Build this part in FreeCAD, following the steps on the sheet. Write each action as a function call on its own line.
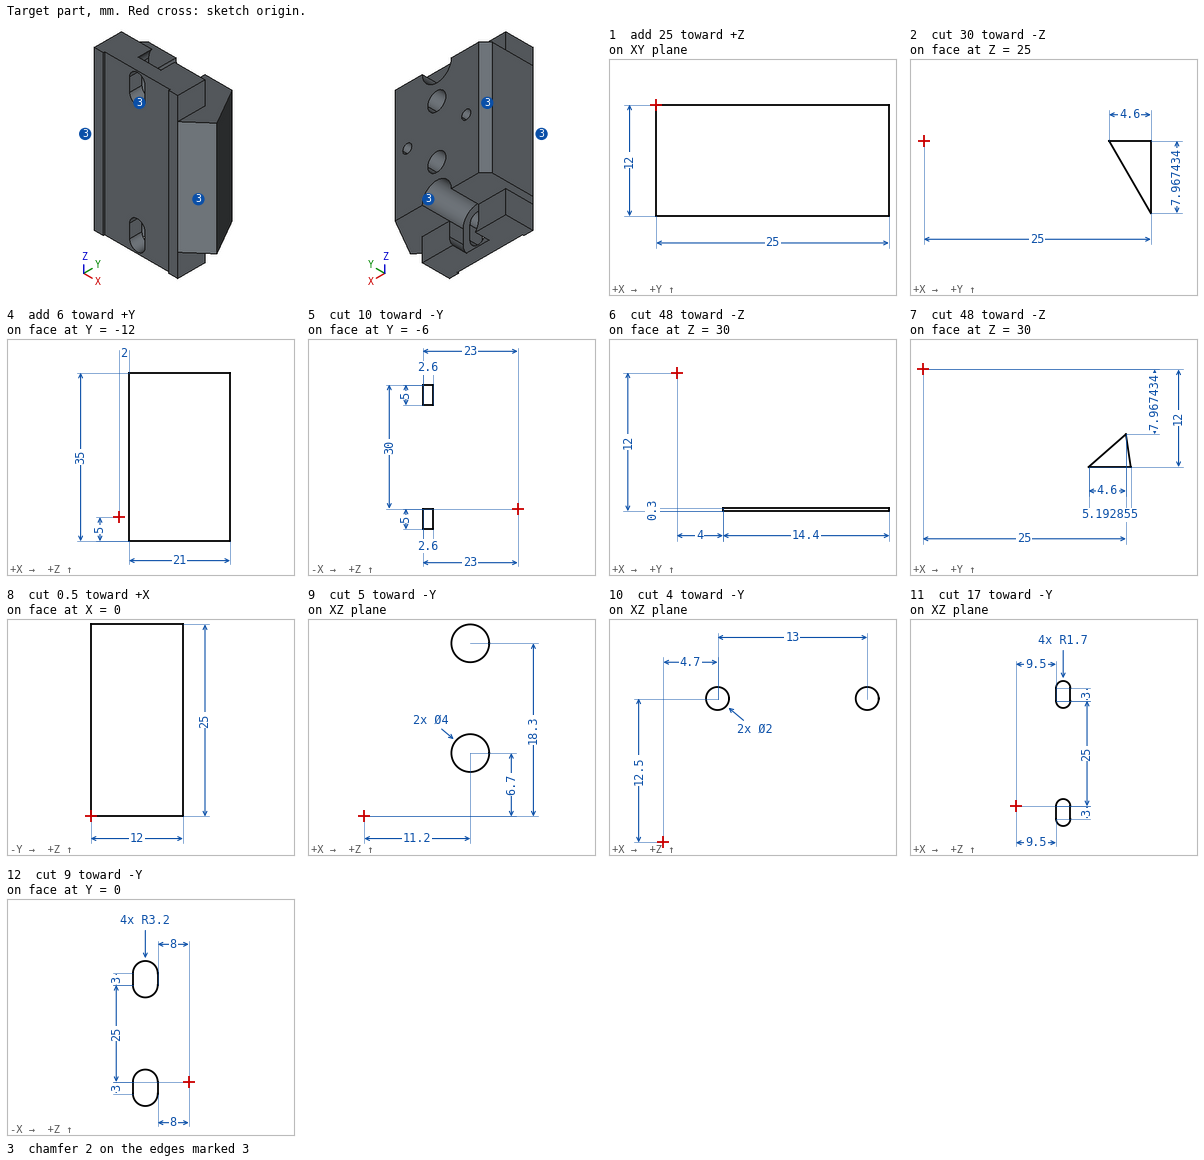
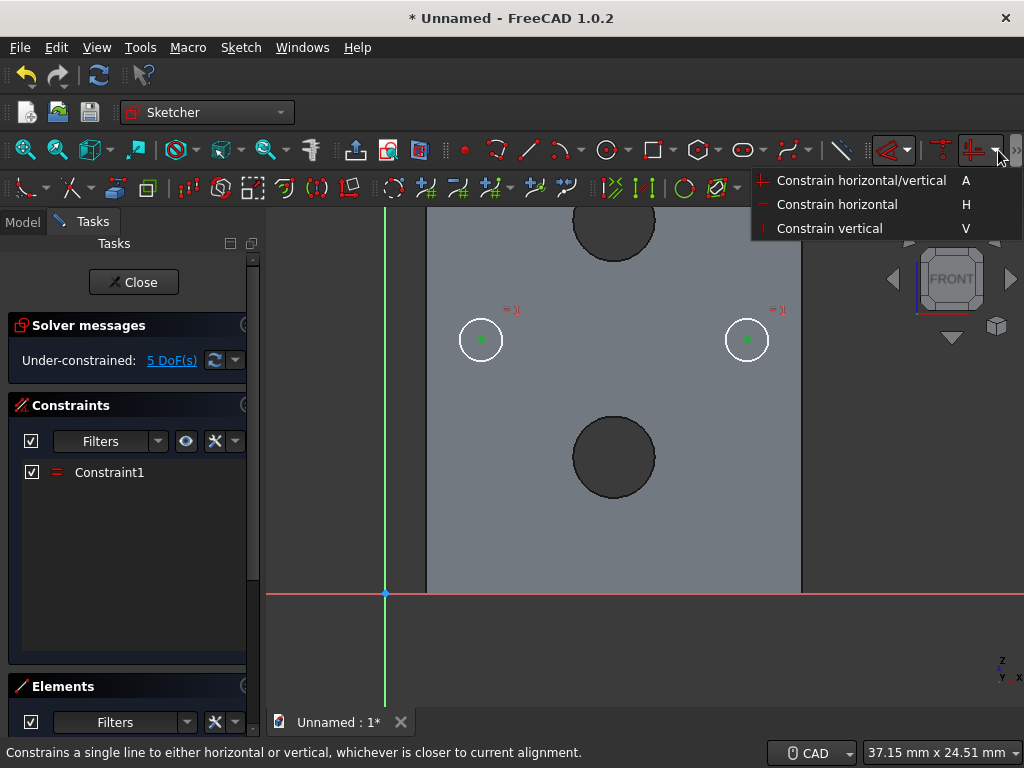
click(887, 204)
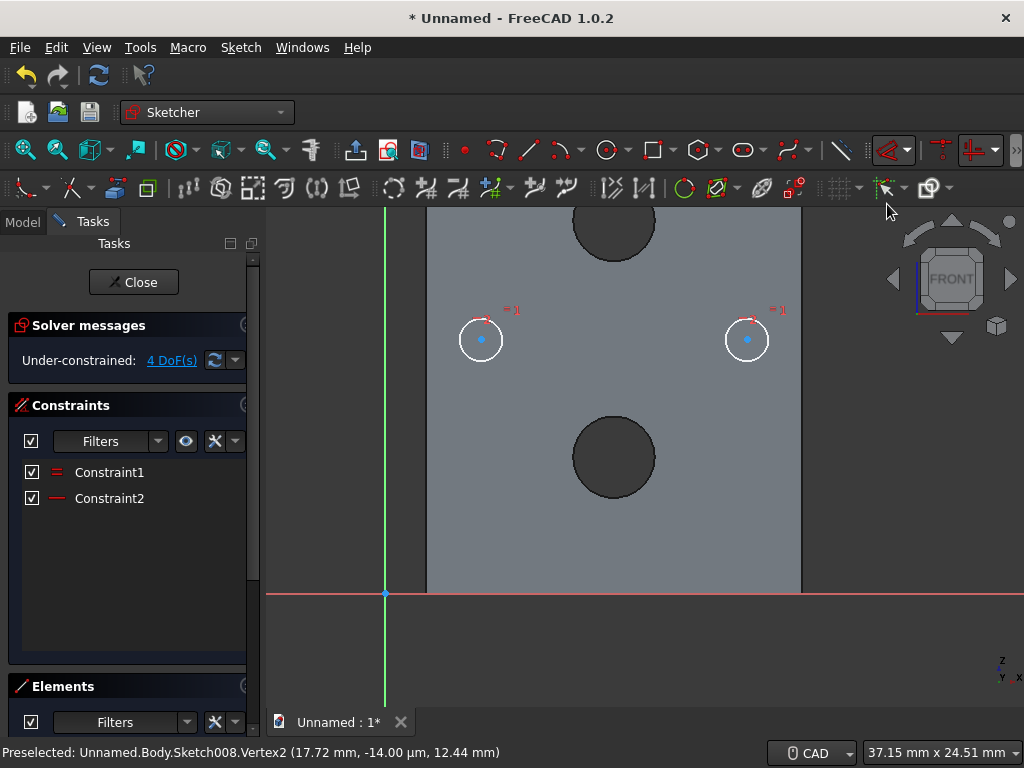
click(496, 325)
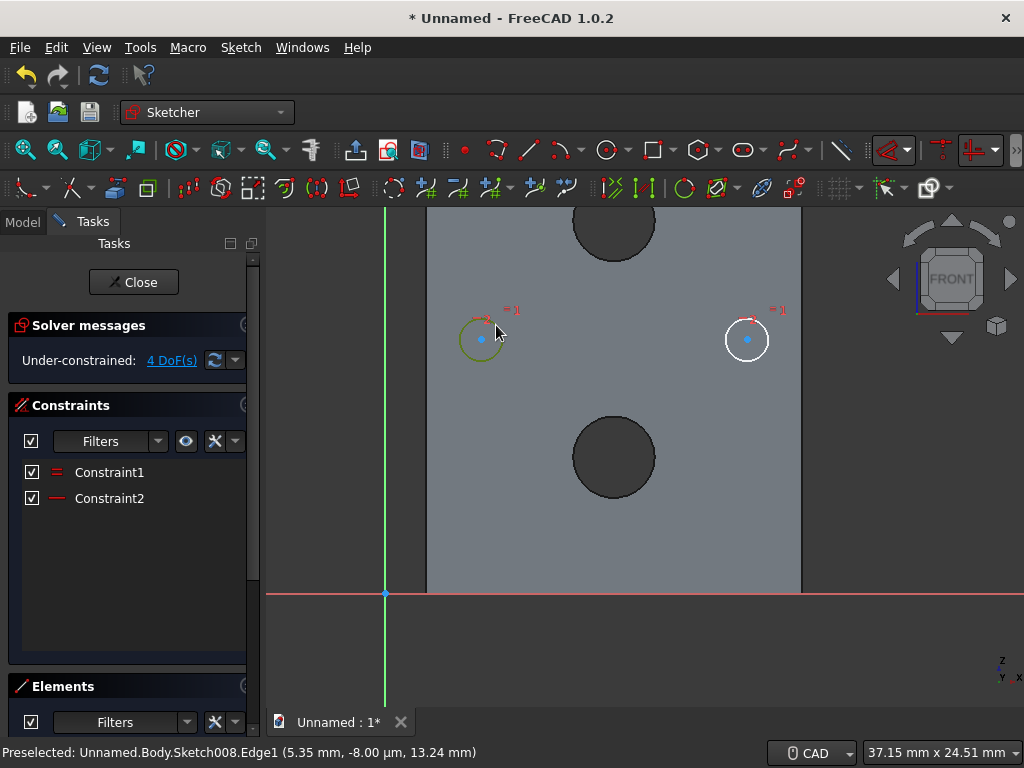
click(910, 150)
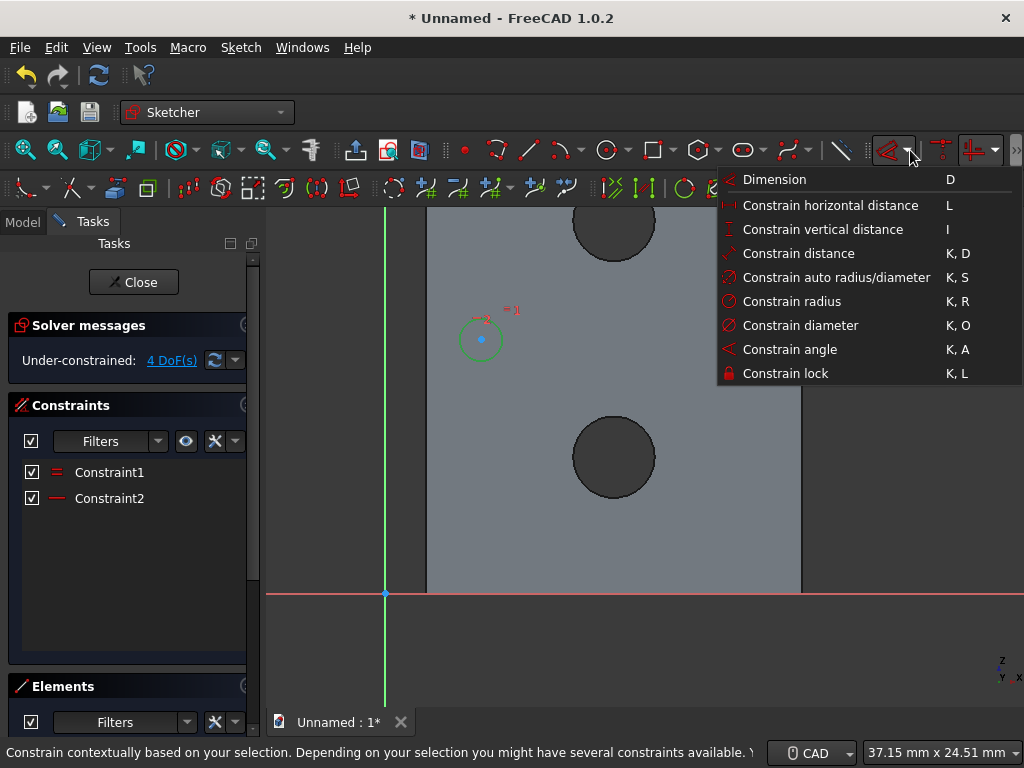
click(870, 325)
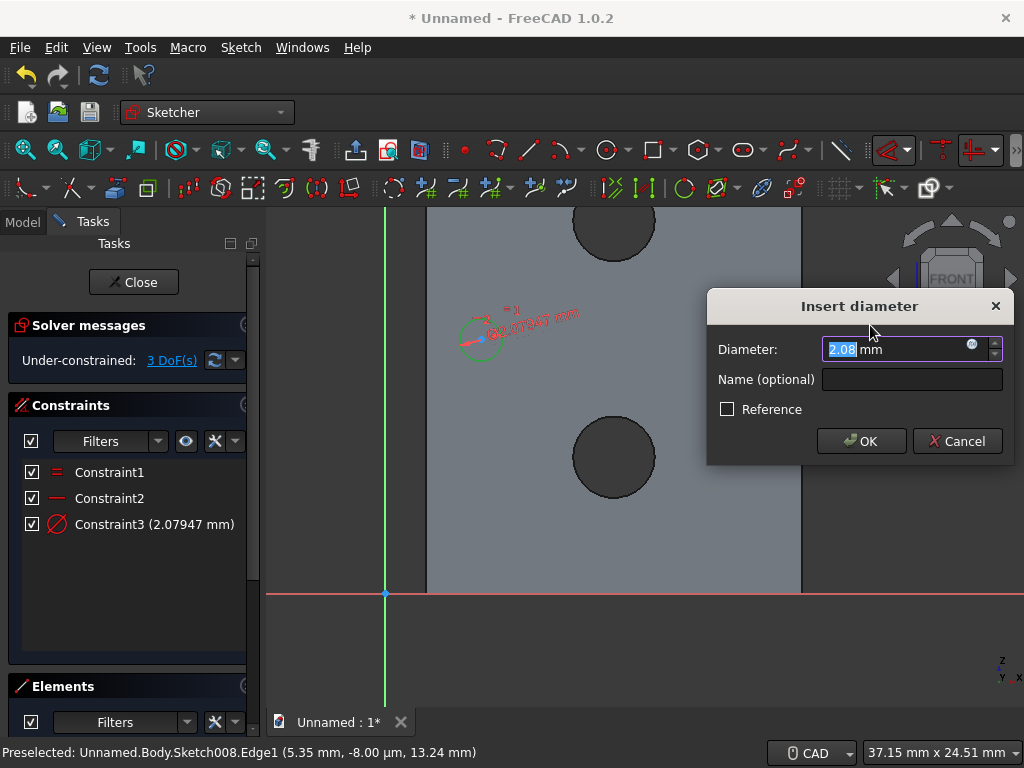
text(2)
key(Return)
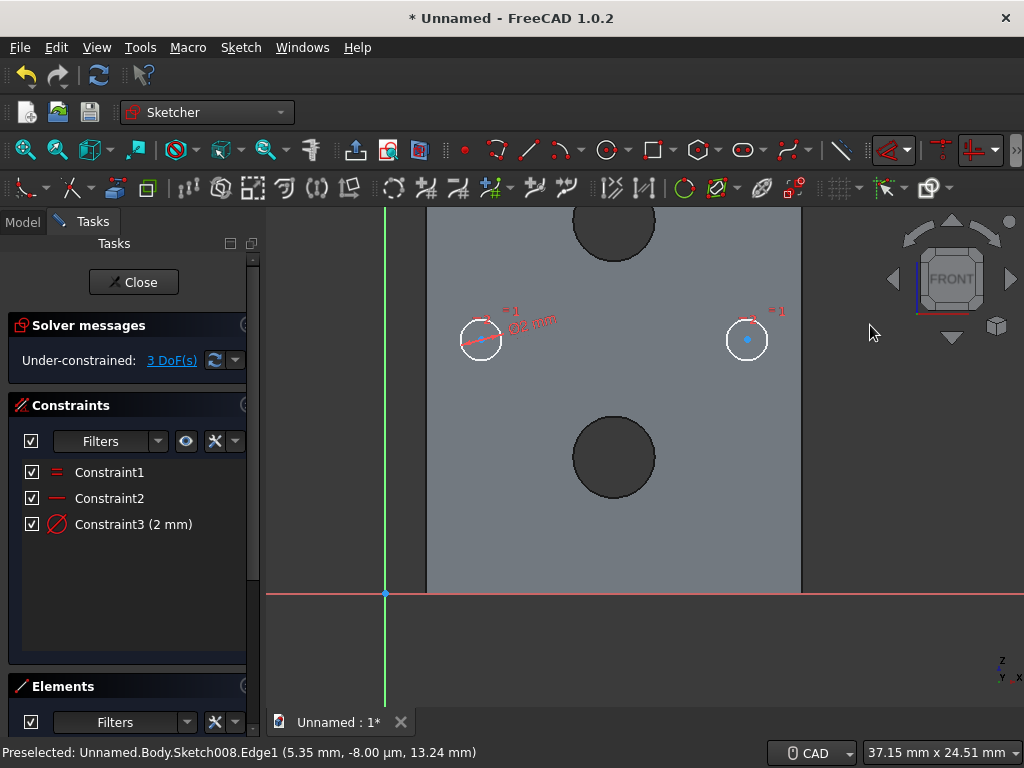
click(481, 340)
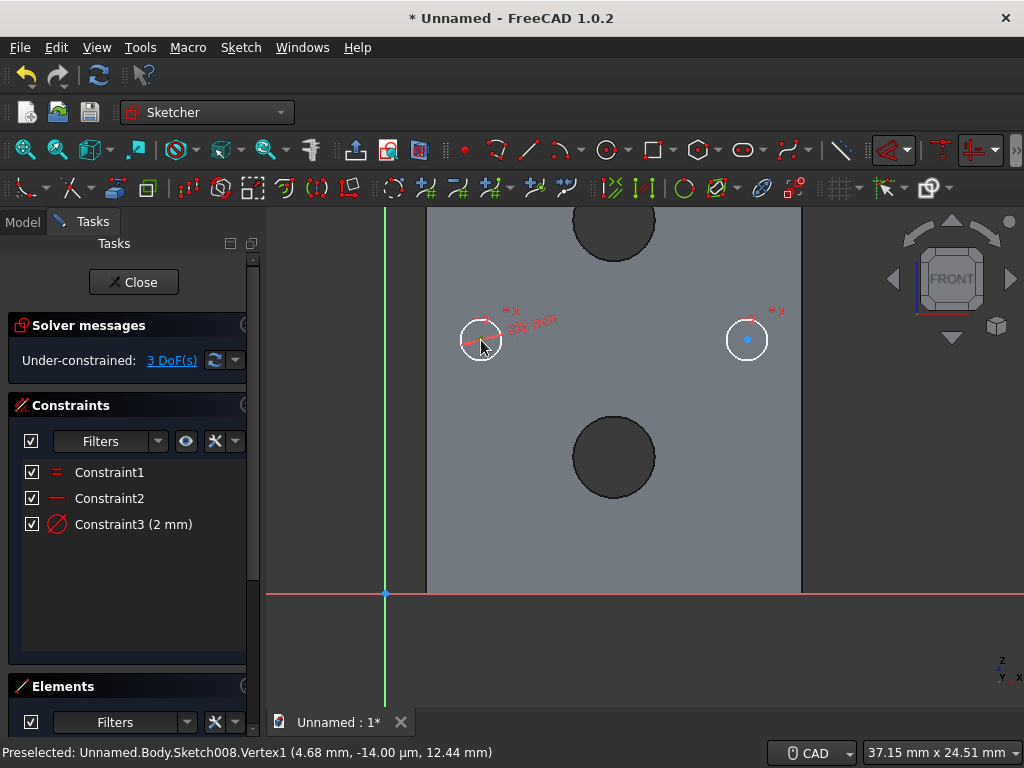
click(910, 150)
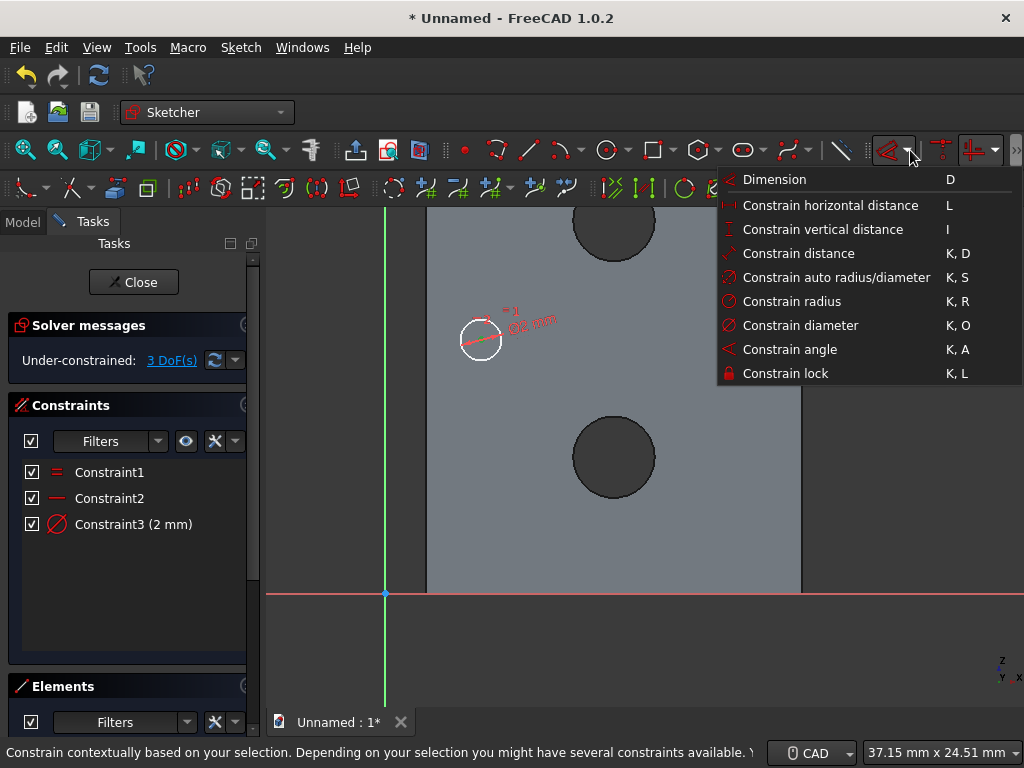
click(870, 205)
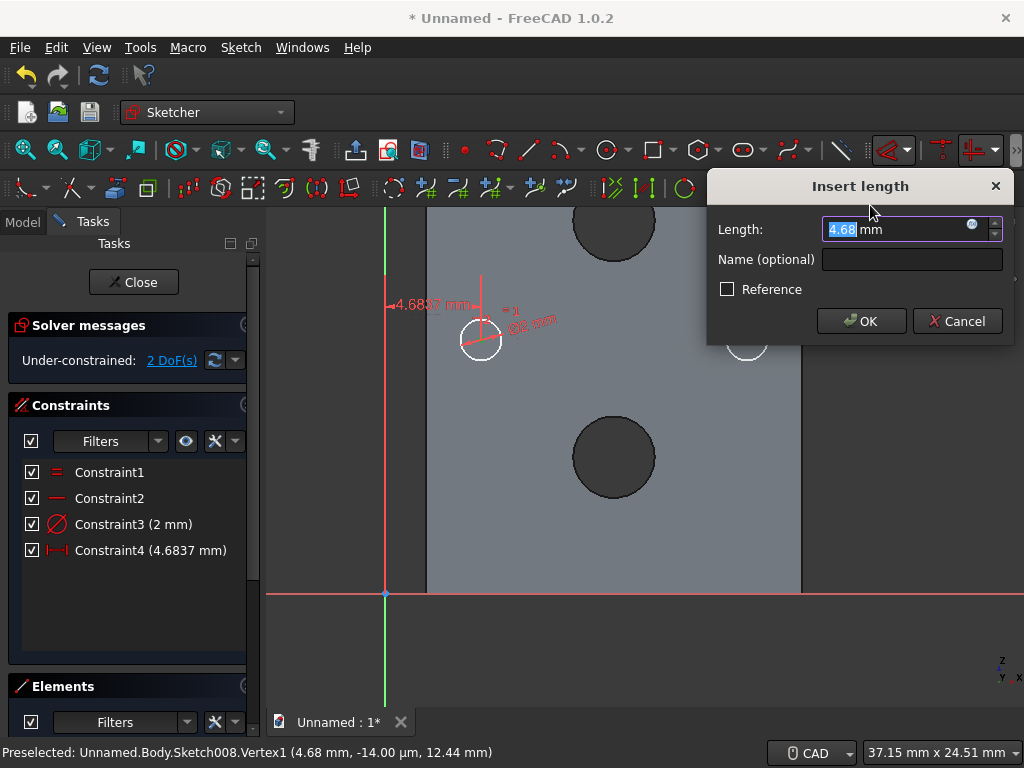
text(4.7)
key(Return)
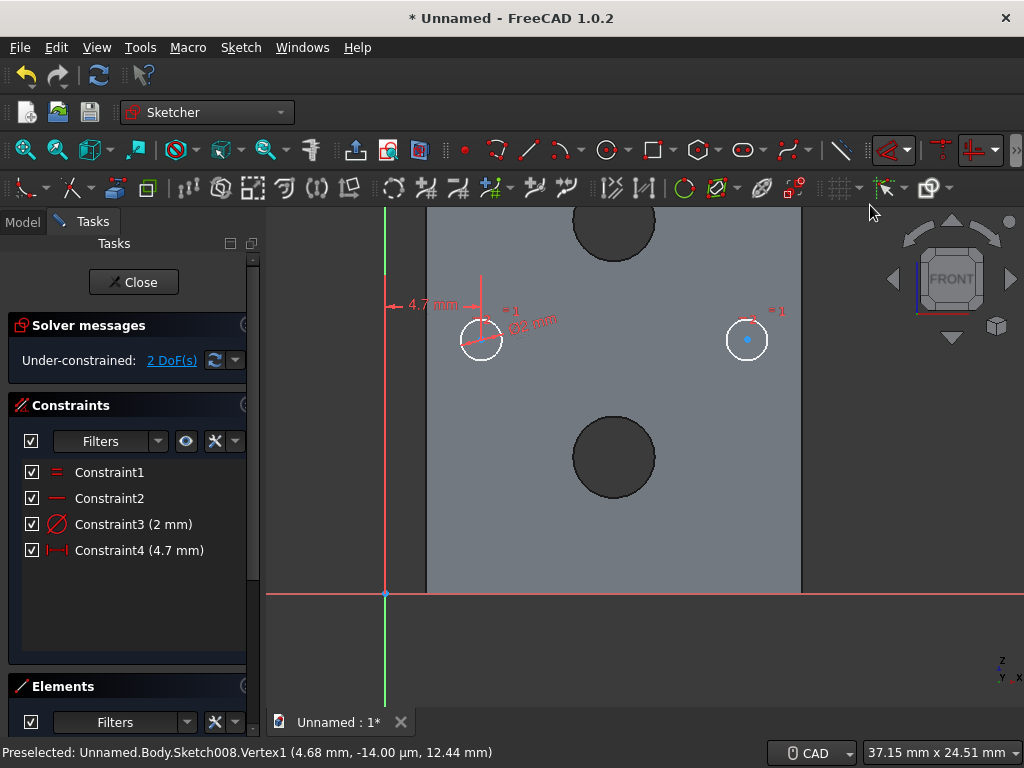
click(481, 340)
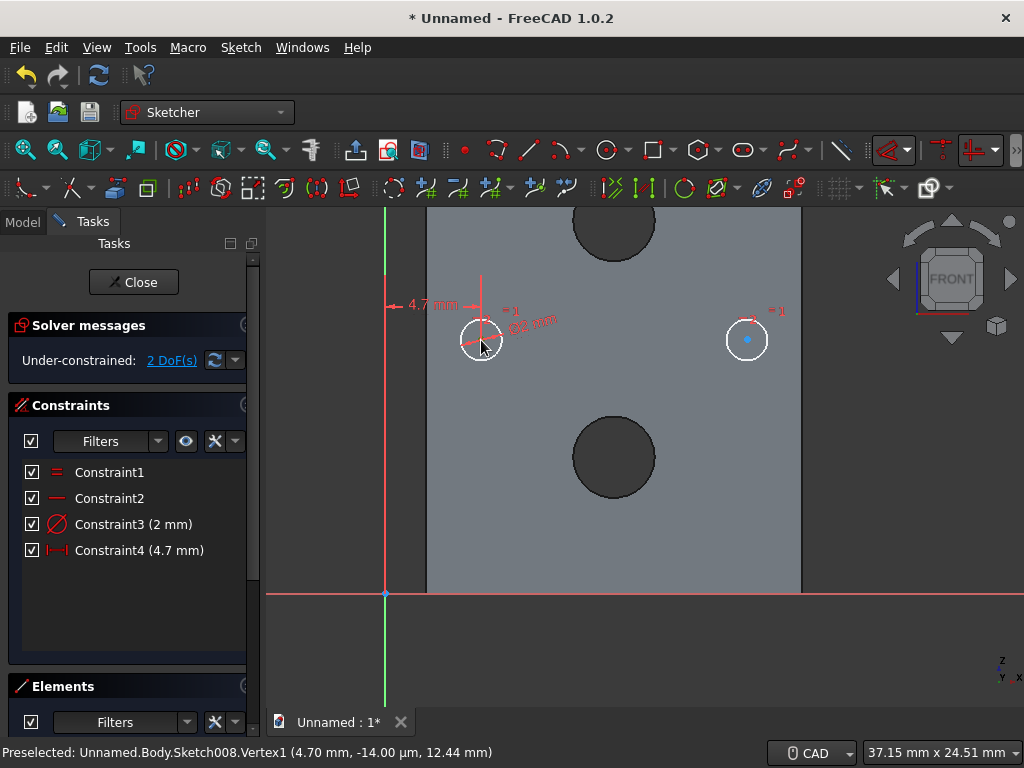
click(747, 340)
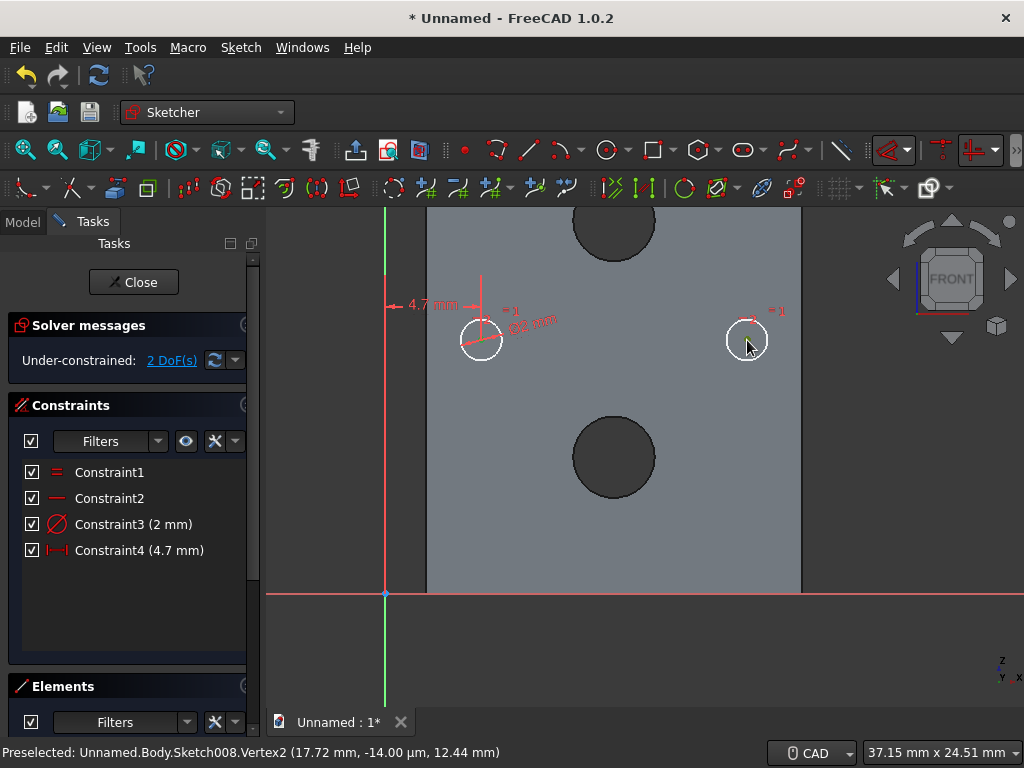
key(l)